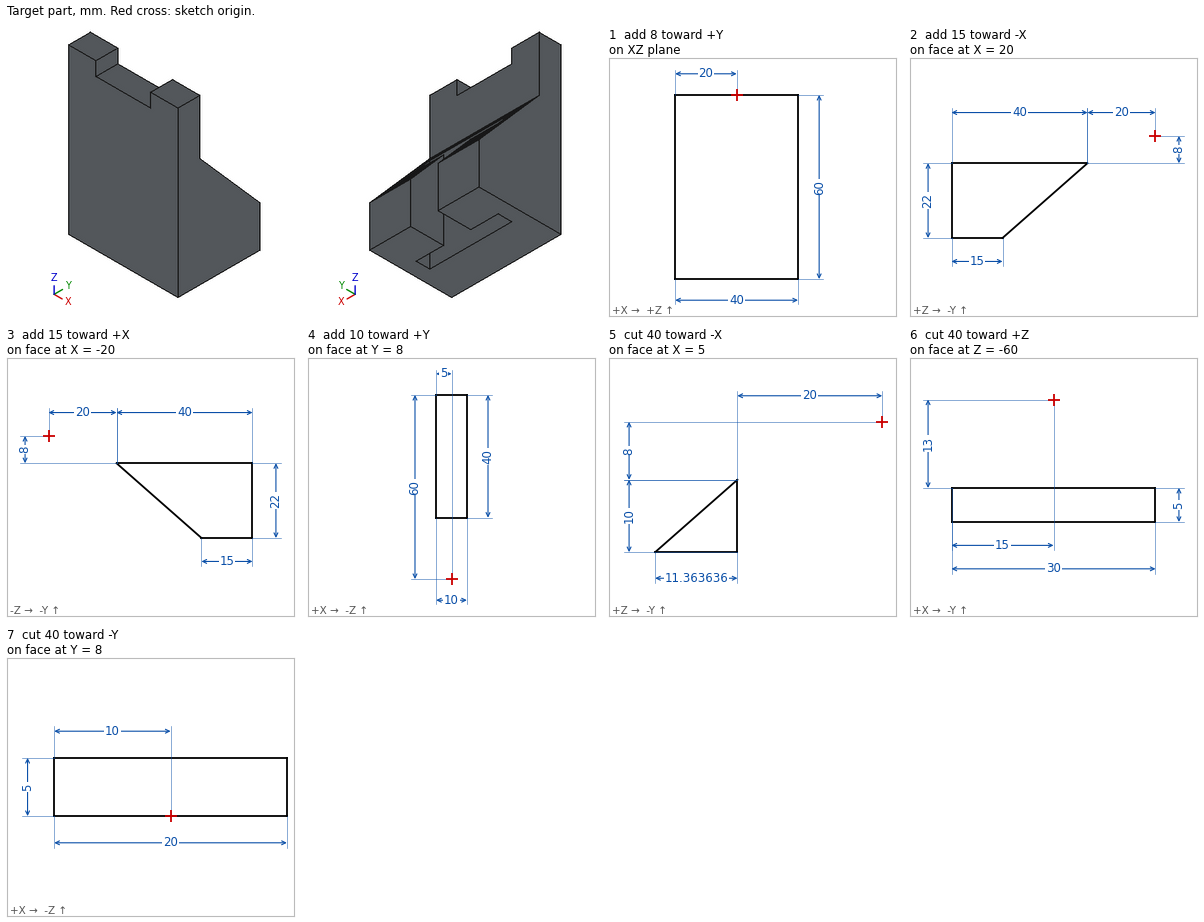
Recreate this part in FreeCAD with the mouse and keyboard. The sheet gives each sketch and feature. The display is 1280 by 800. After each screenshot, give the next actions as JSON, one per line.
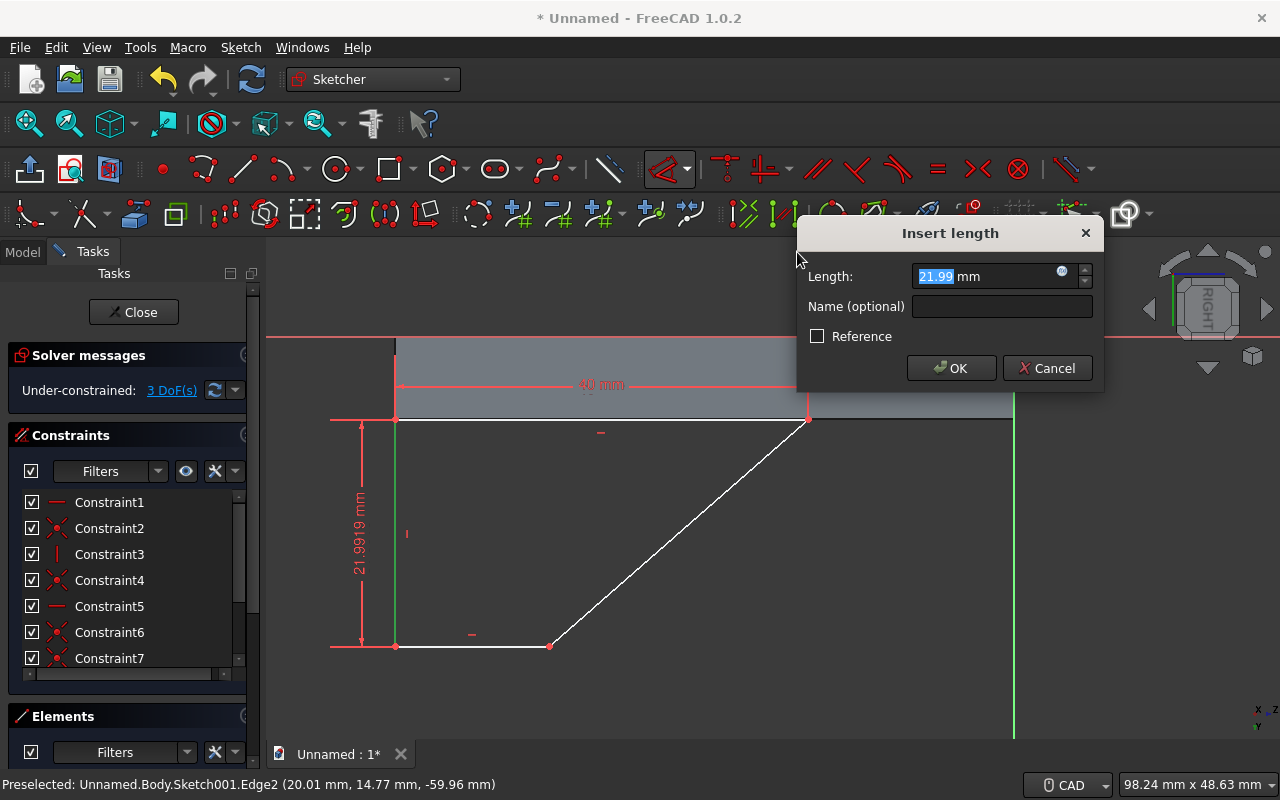
{"action": "type", "text": "22"}
{"action": "key", "text": "Return"}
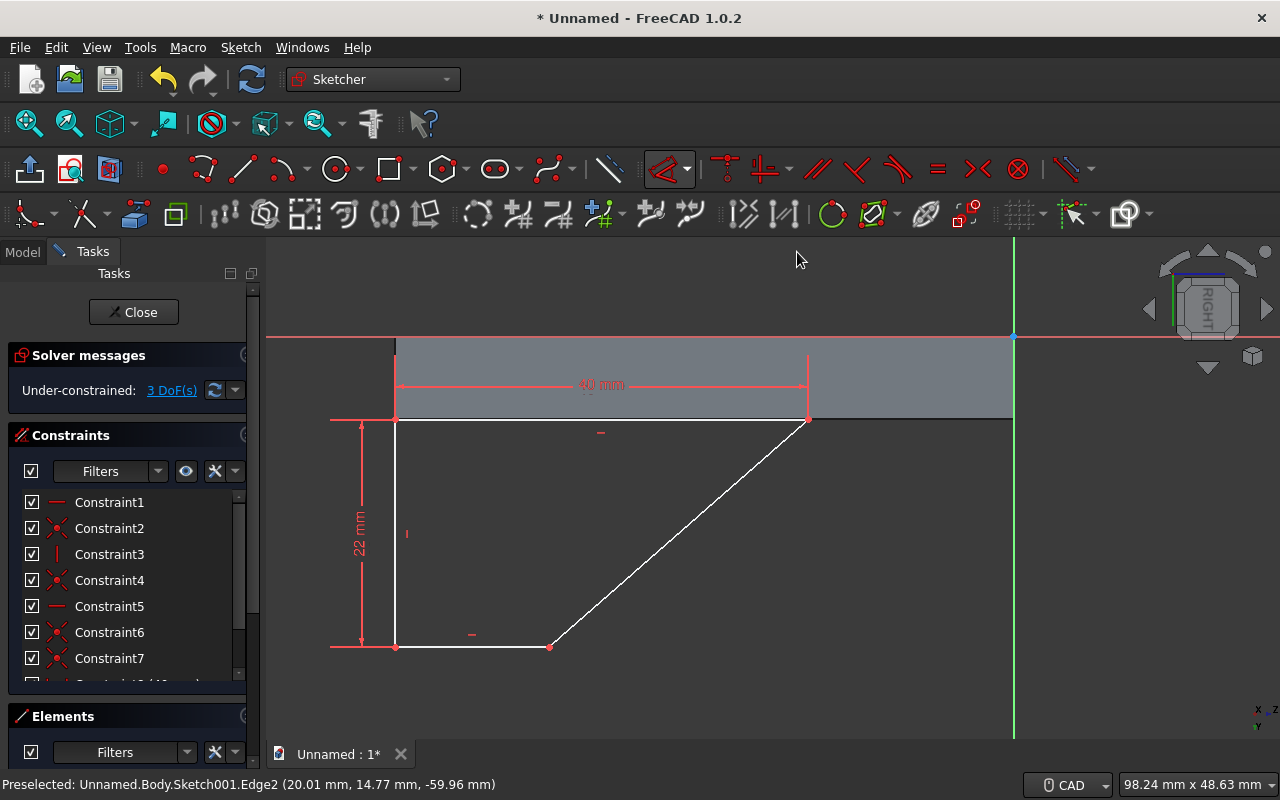
{"action": "left_click", "coordinate": [441, 647]}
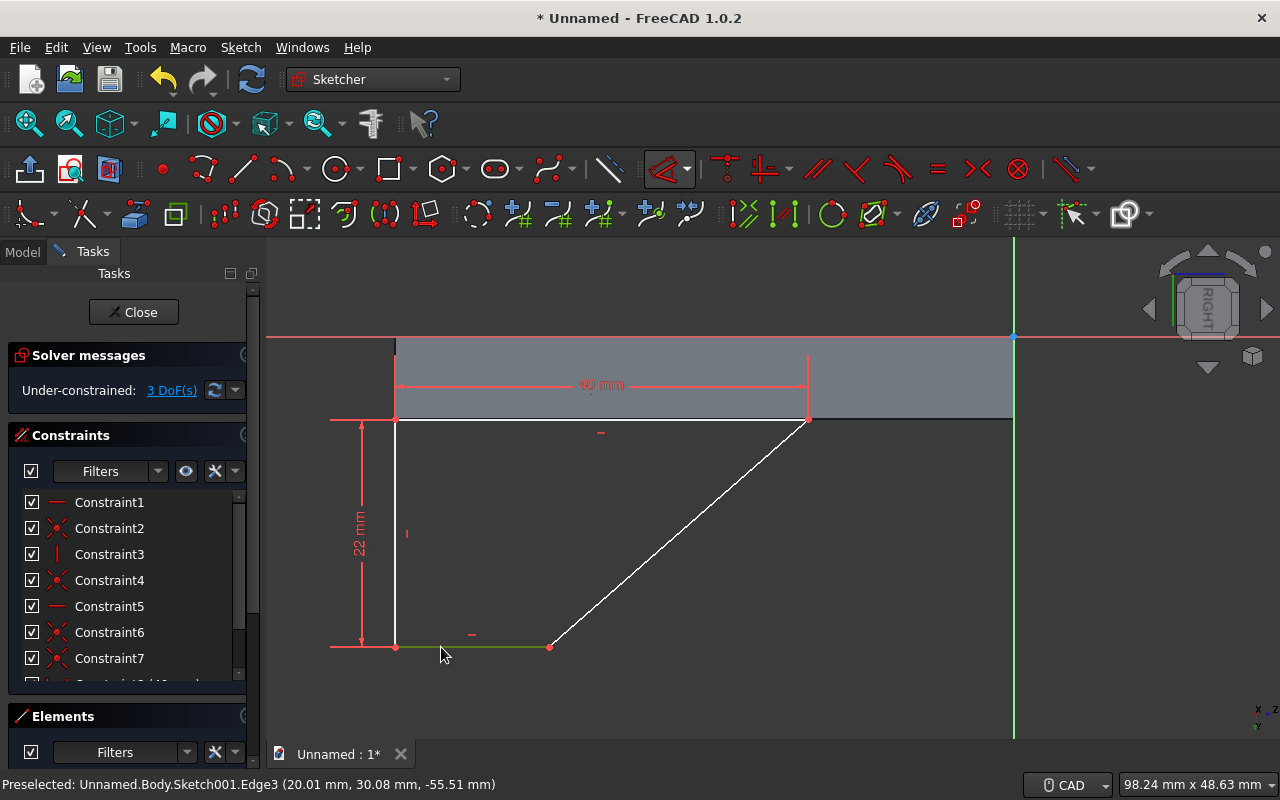
{"action": "left_click", "coordinate": [690, 170]}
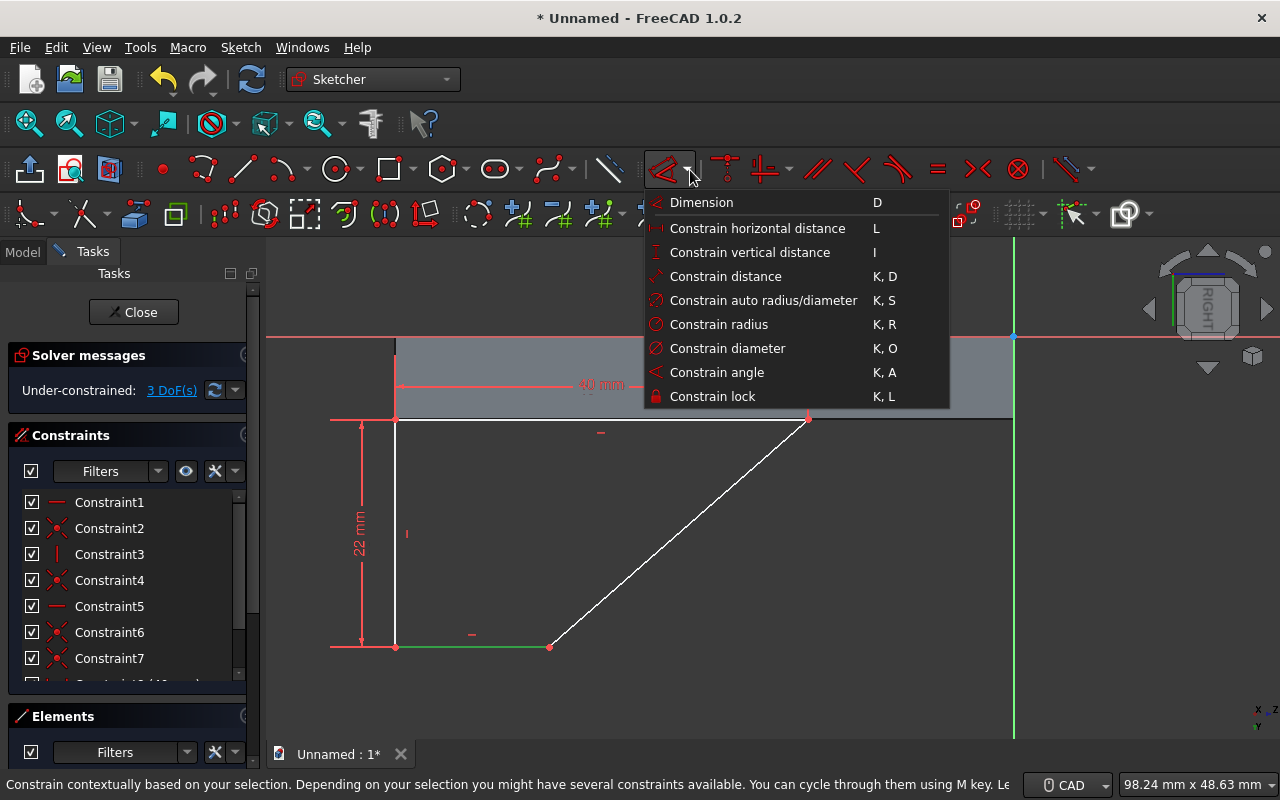
{"action": "left_click", "coordinate": [797, 228]}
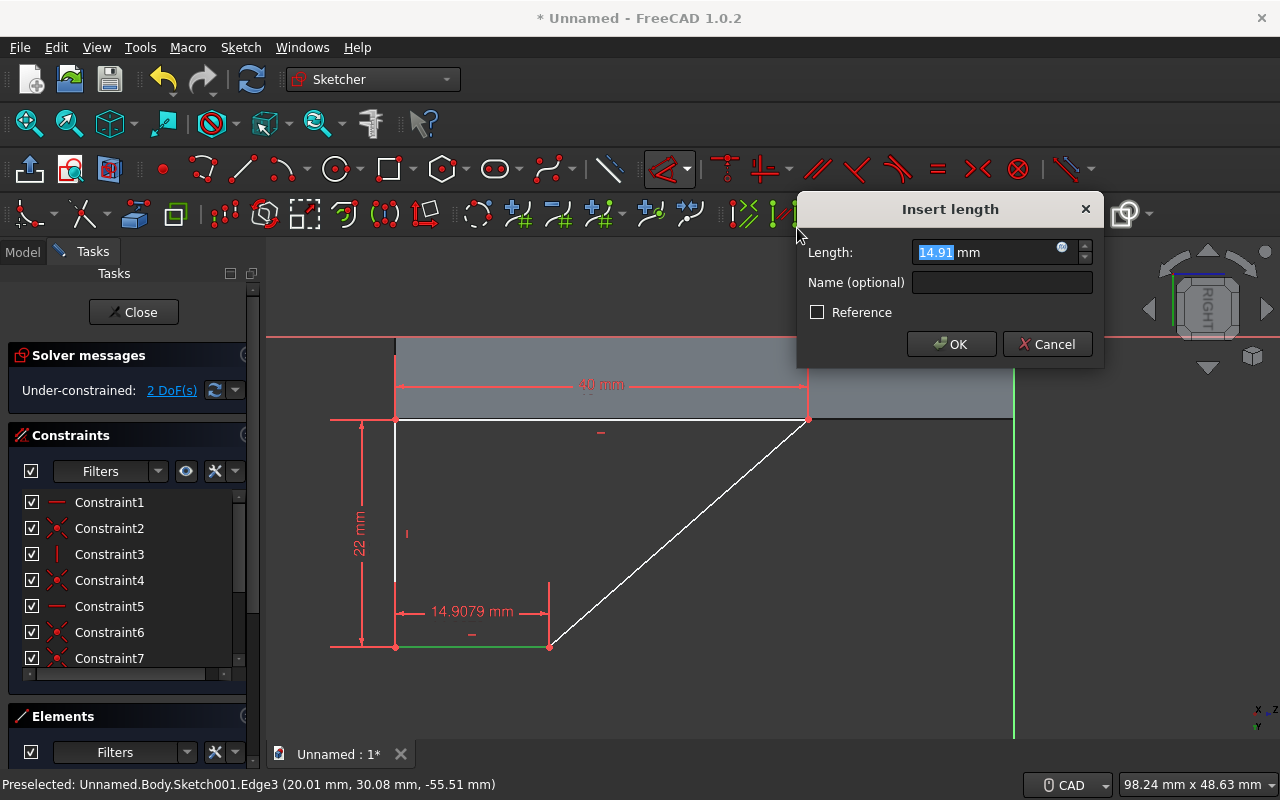
{"action": "type", "text": "15"}
{"action": "key", "text": "Return"}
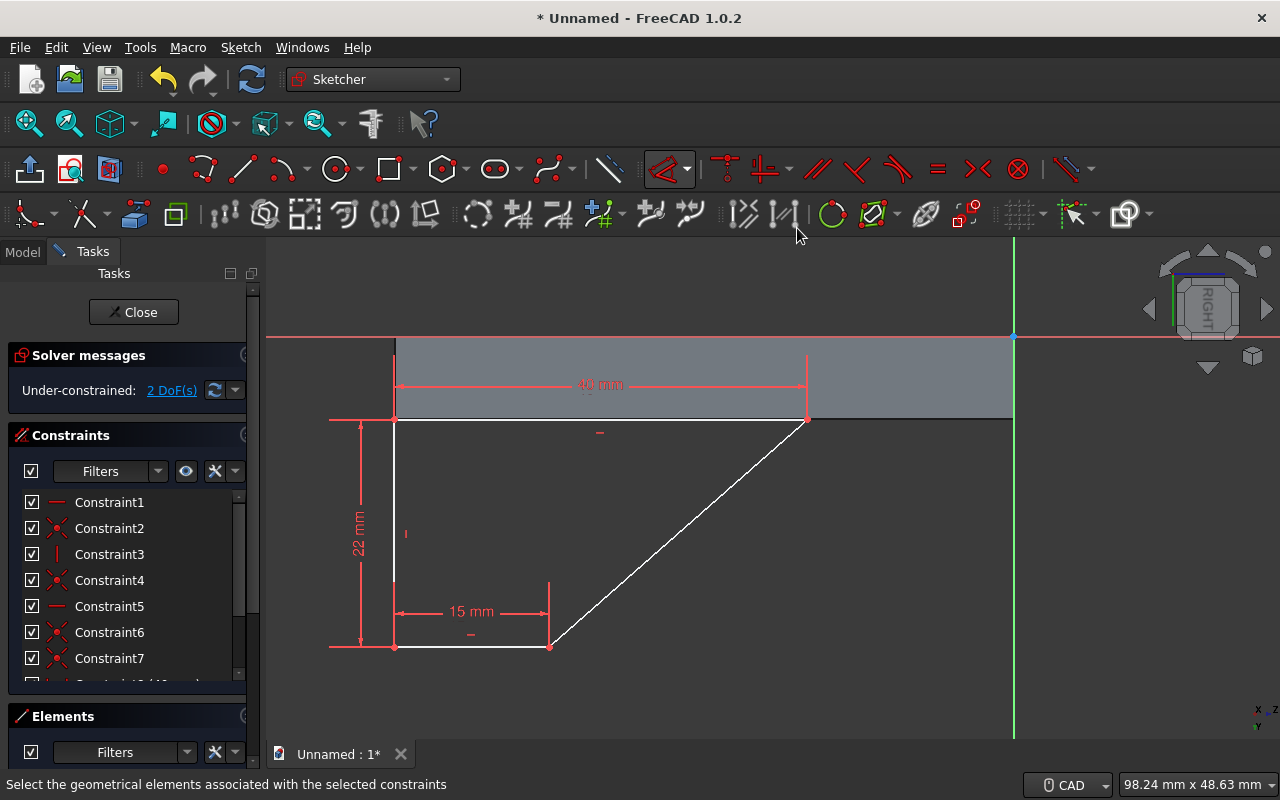
{"action": "left_click", "coordinate": [807, 420]}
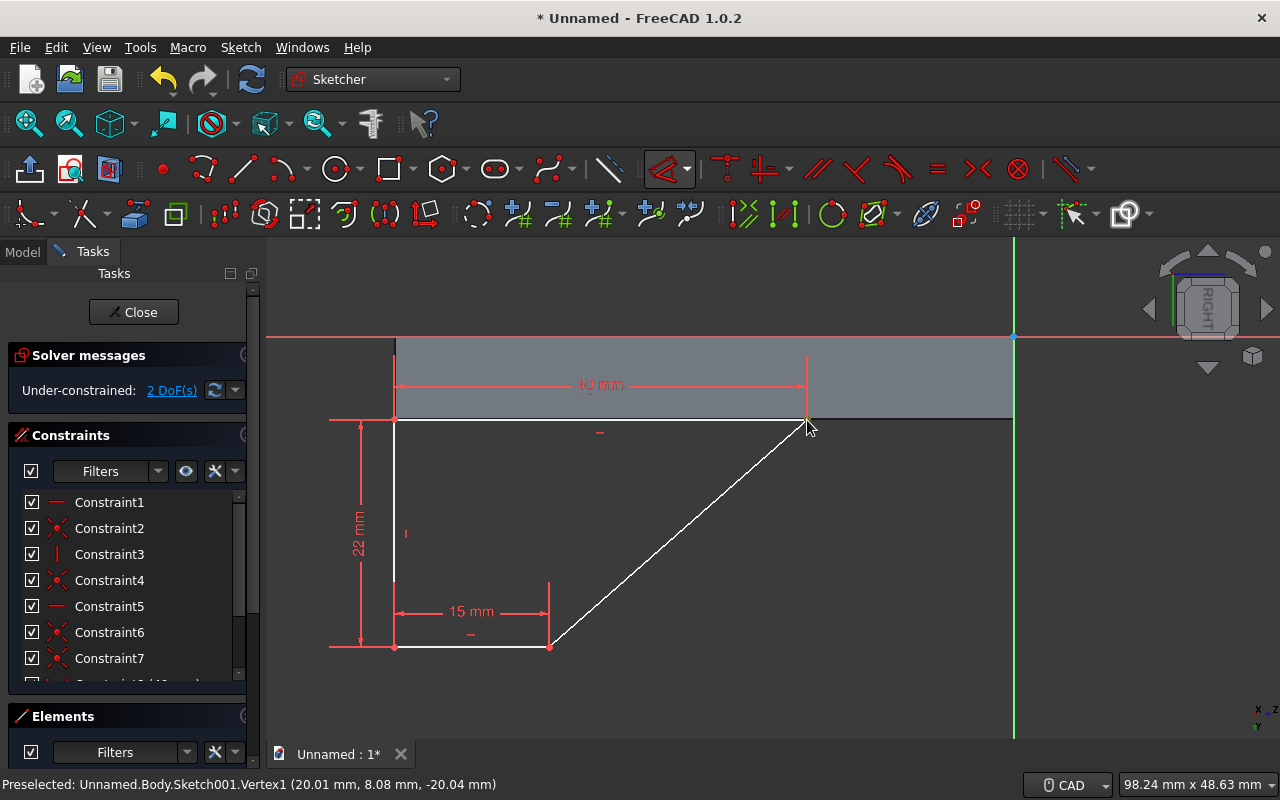
{"action": "key", "text": "i"}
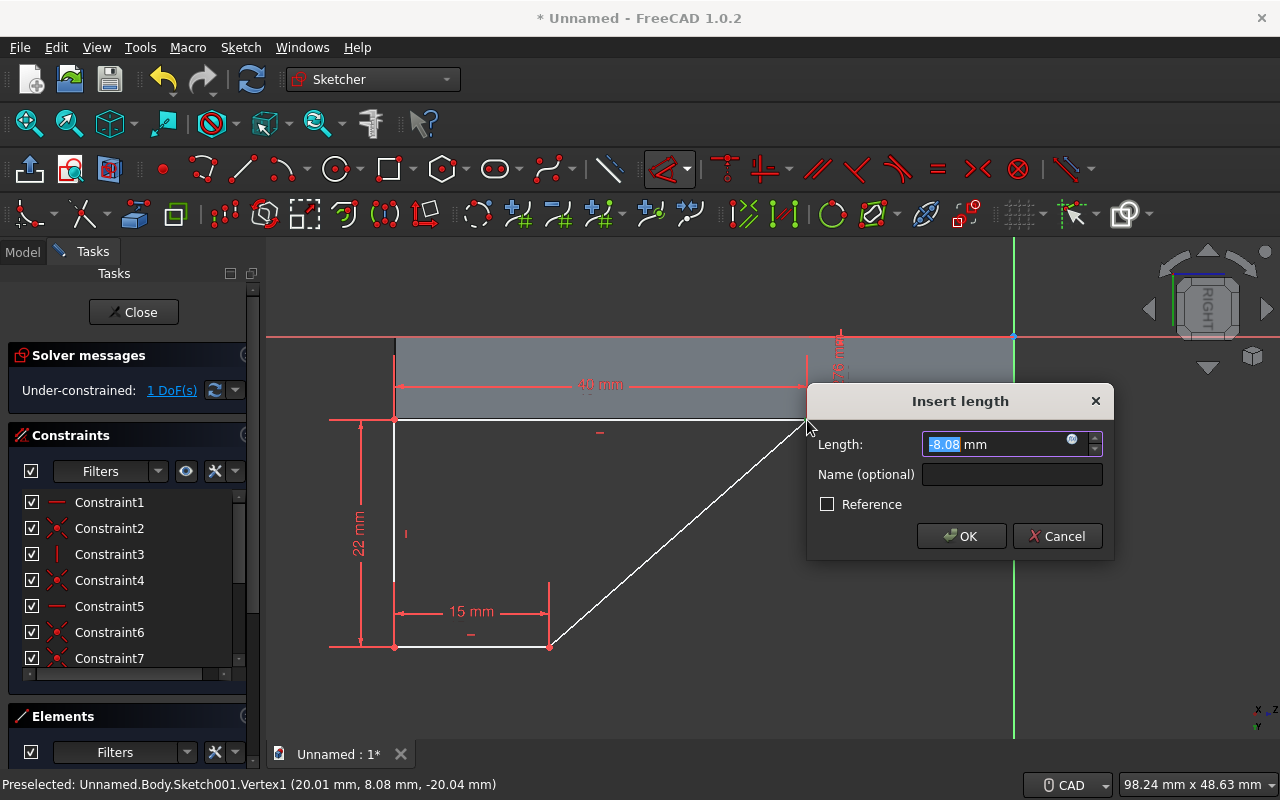
{"action": "type", "text": "-8"}
{"action": "key", "text": "Return"}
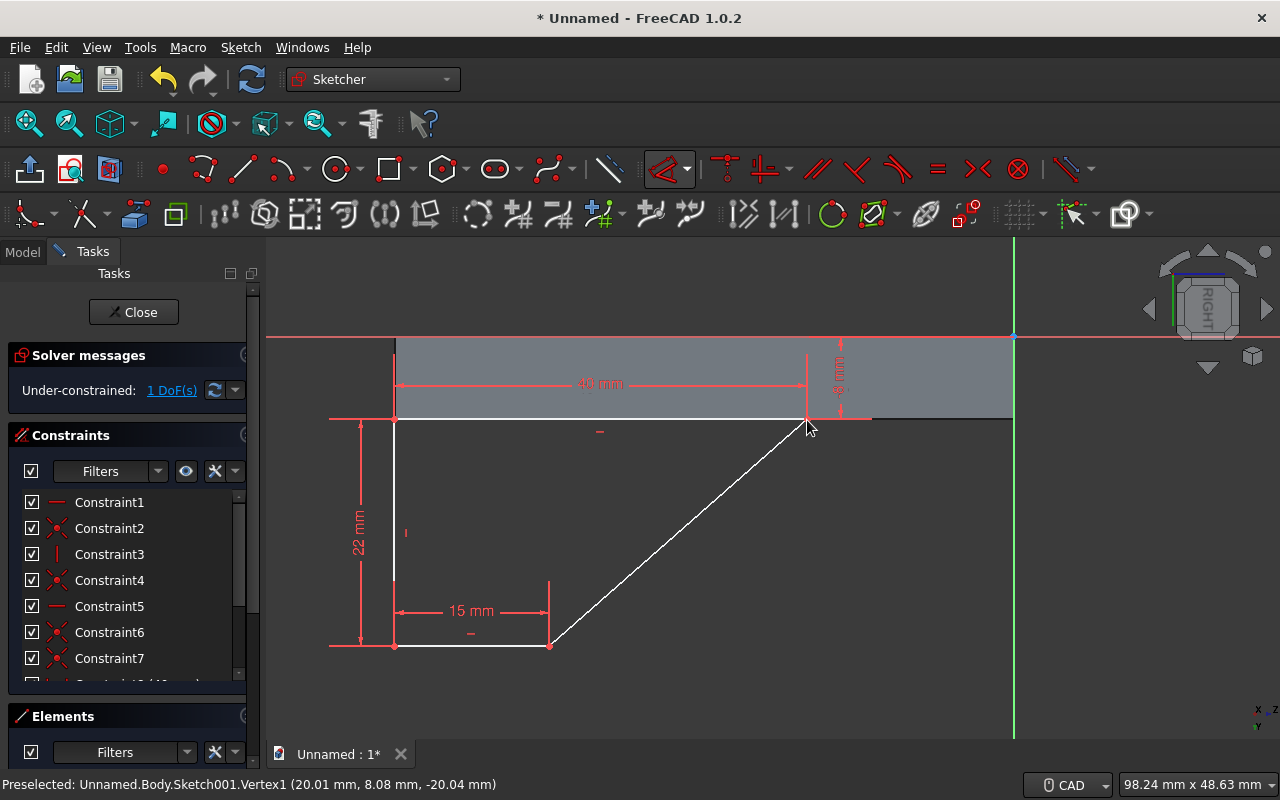
{"action": "left_click", "coordinate": [807, 419]}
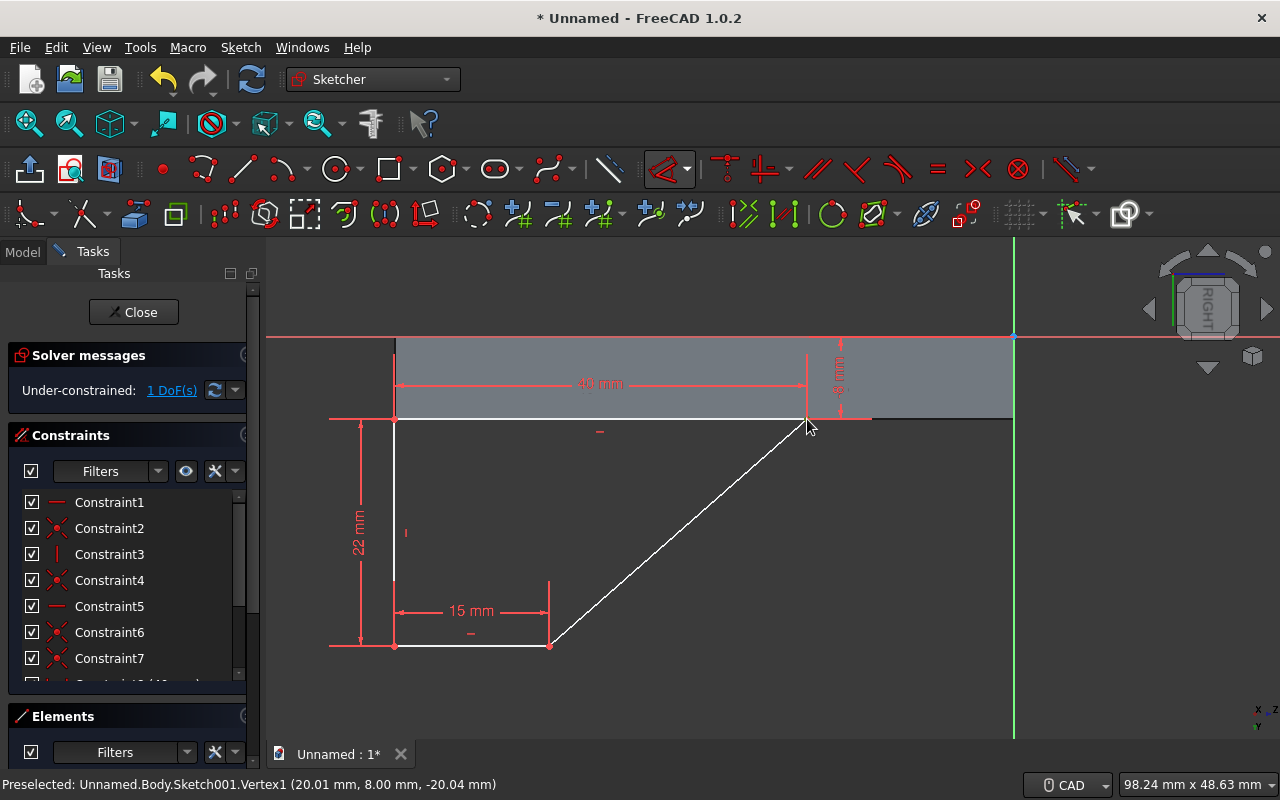
{"action": "left_click", "coordinate": [690, 170]}